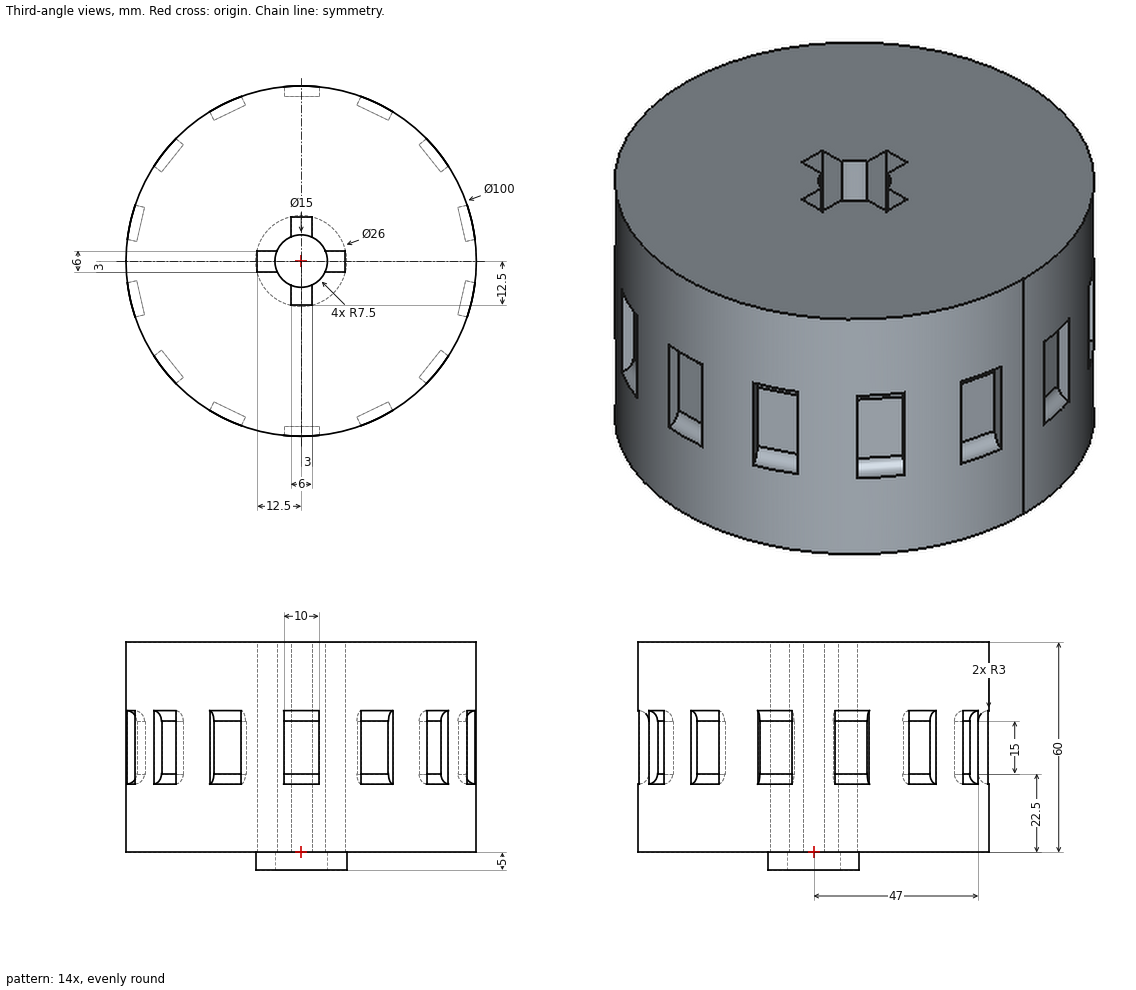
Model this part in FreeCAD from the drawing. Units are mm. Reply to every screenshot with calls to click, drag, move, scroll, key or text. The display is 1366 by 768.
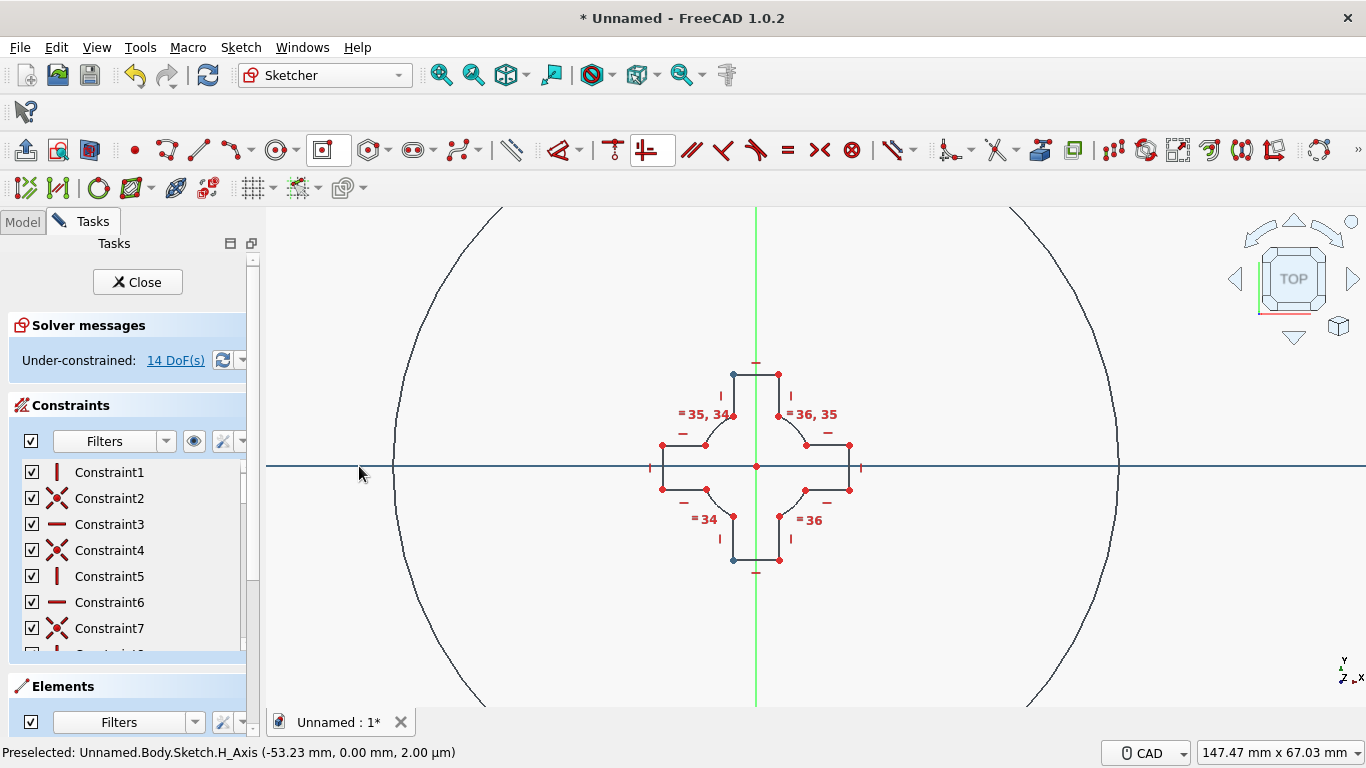
click(820, 150)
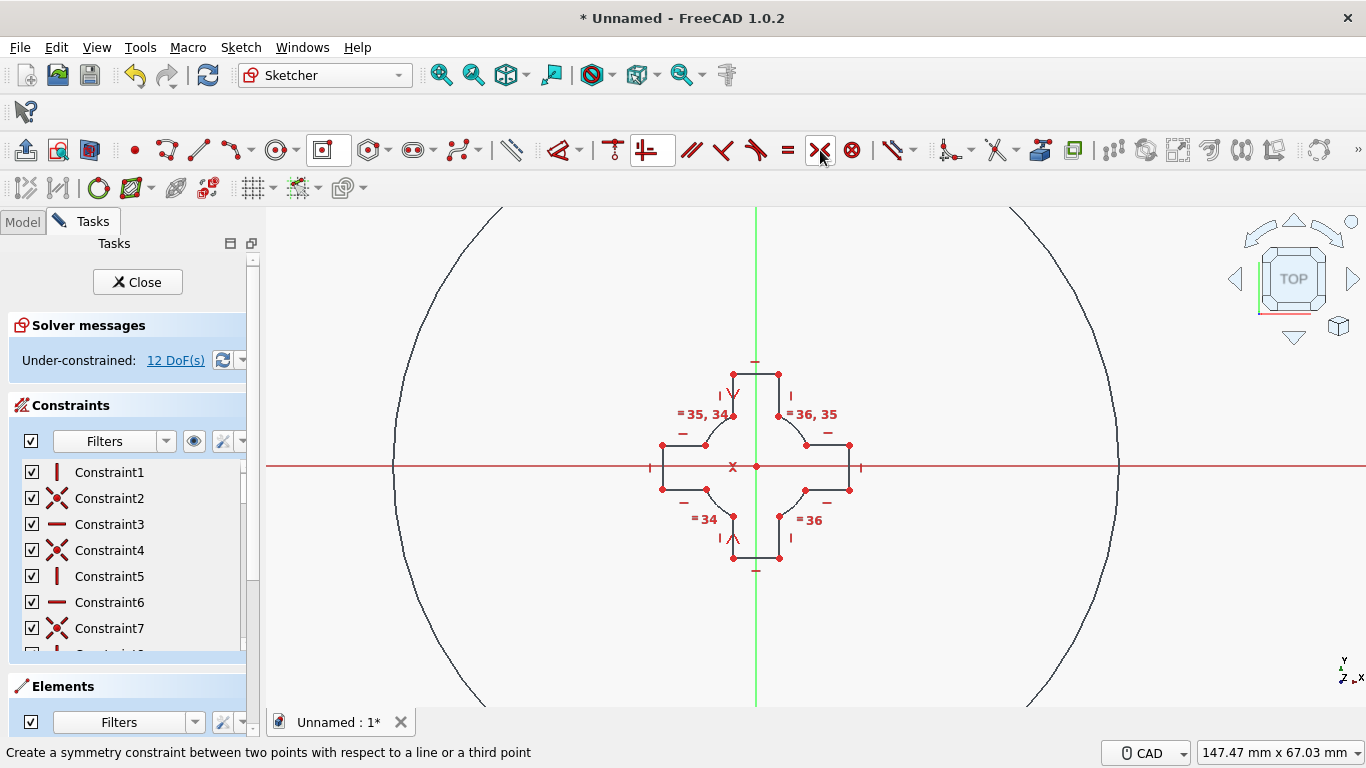
click(663, 446)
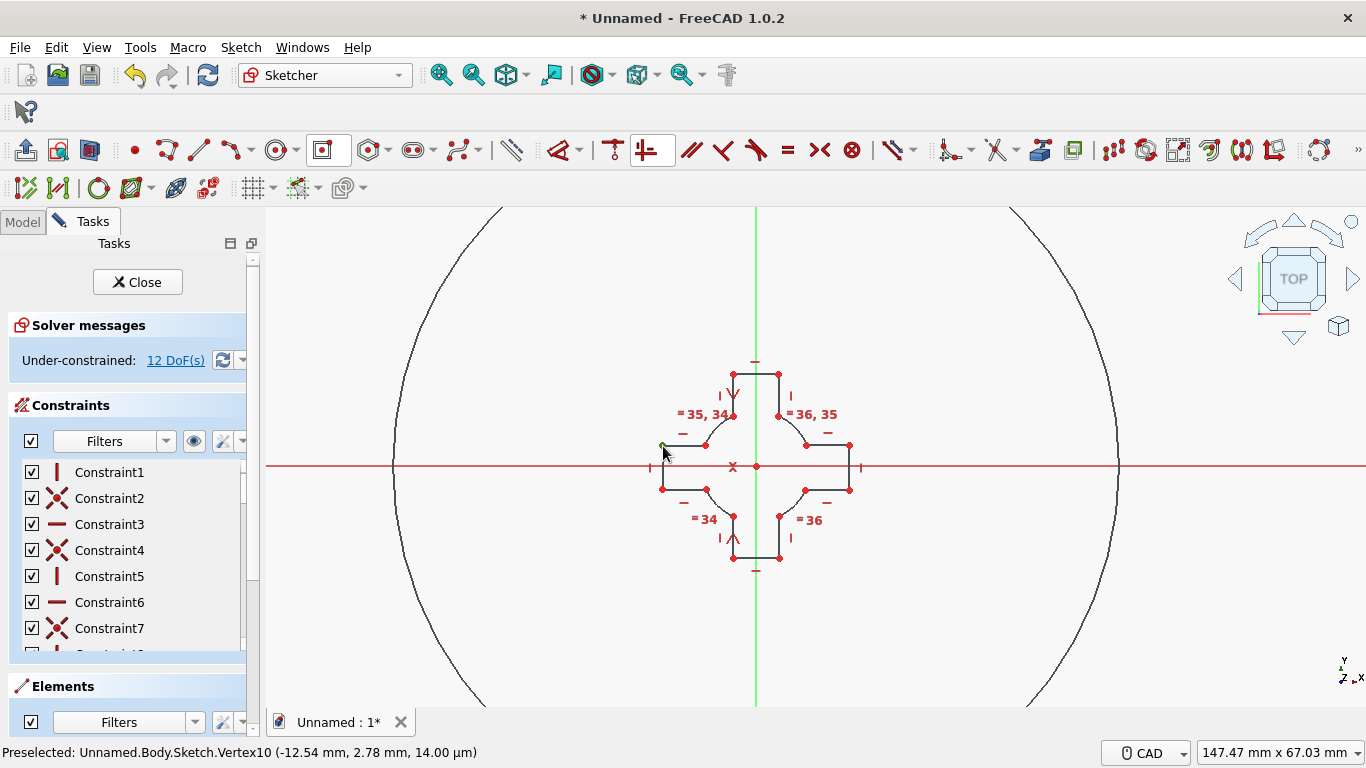
click(849, 445)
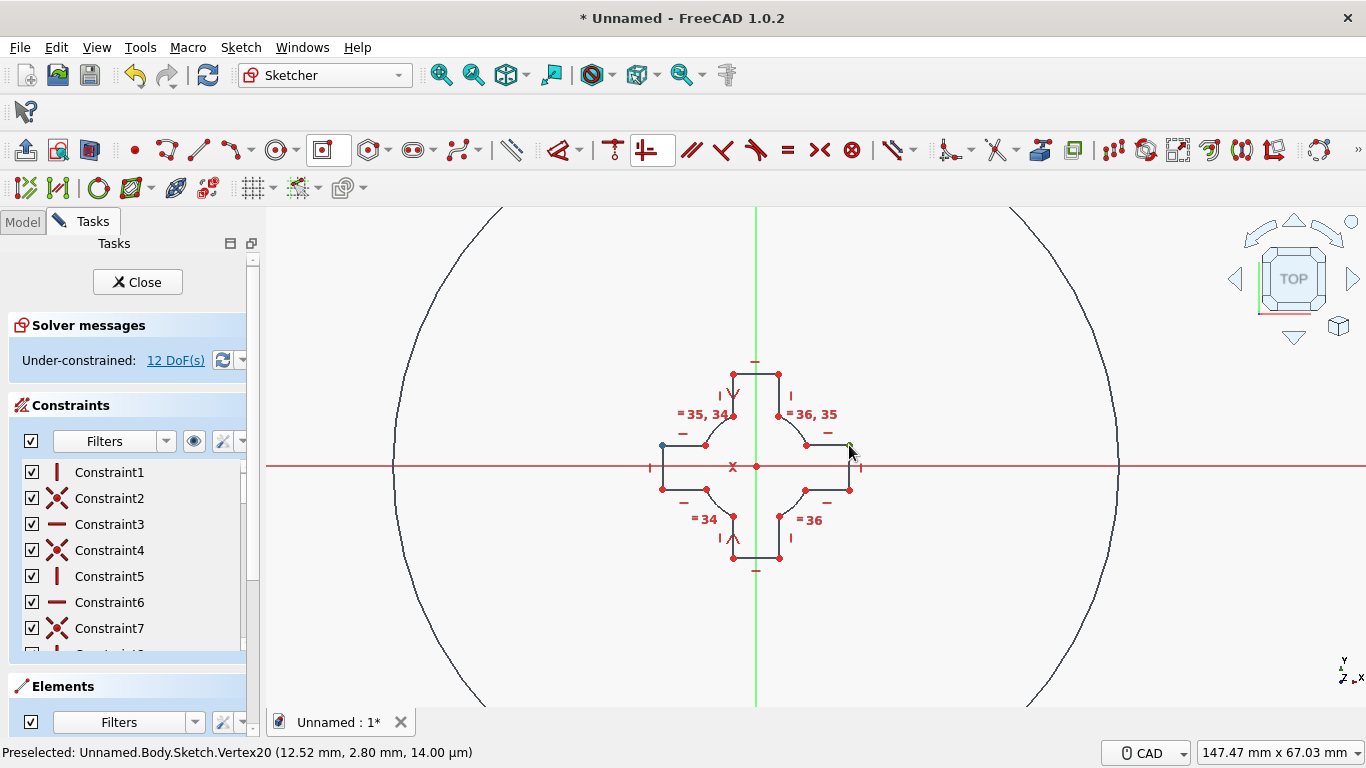
click(756, 647)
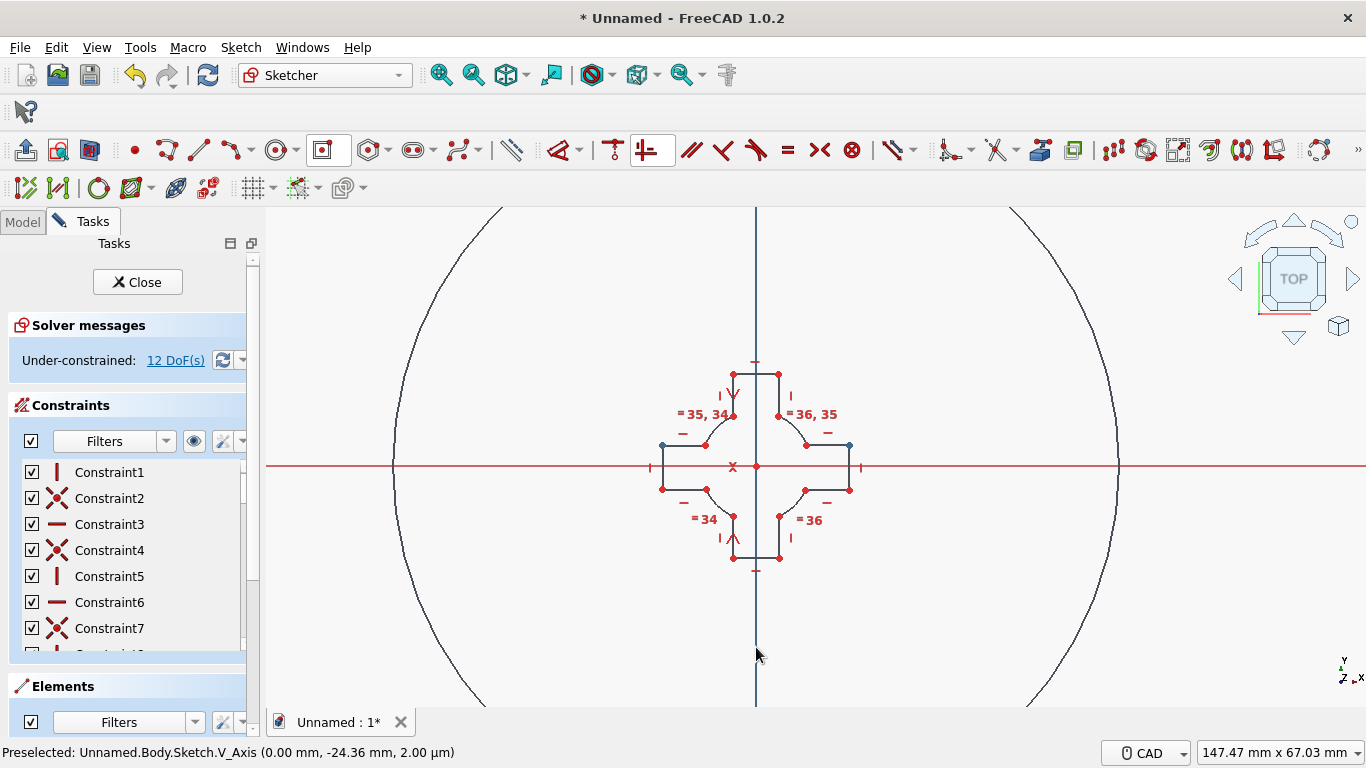
key(s)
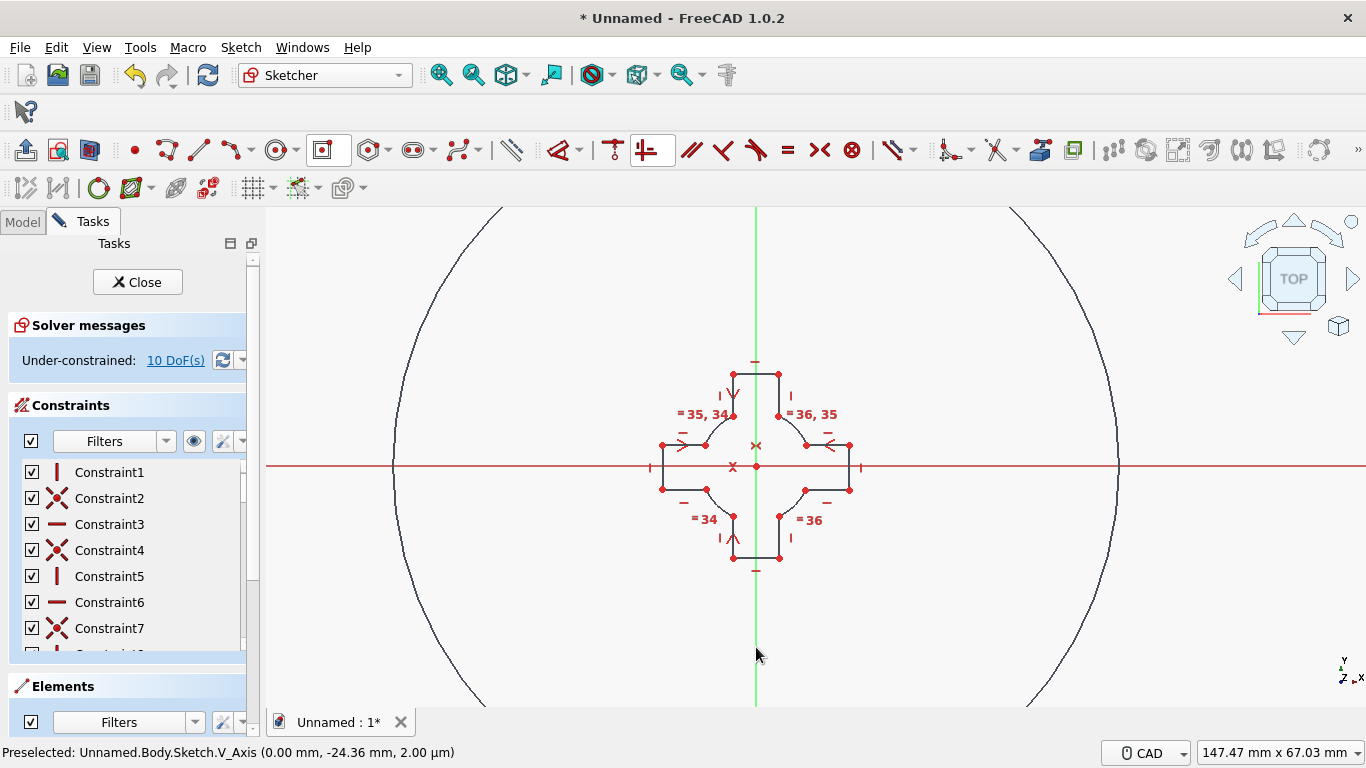
key(d)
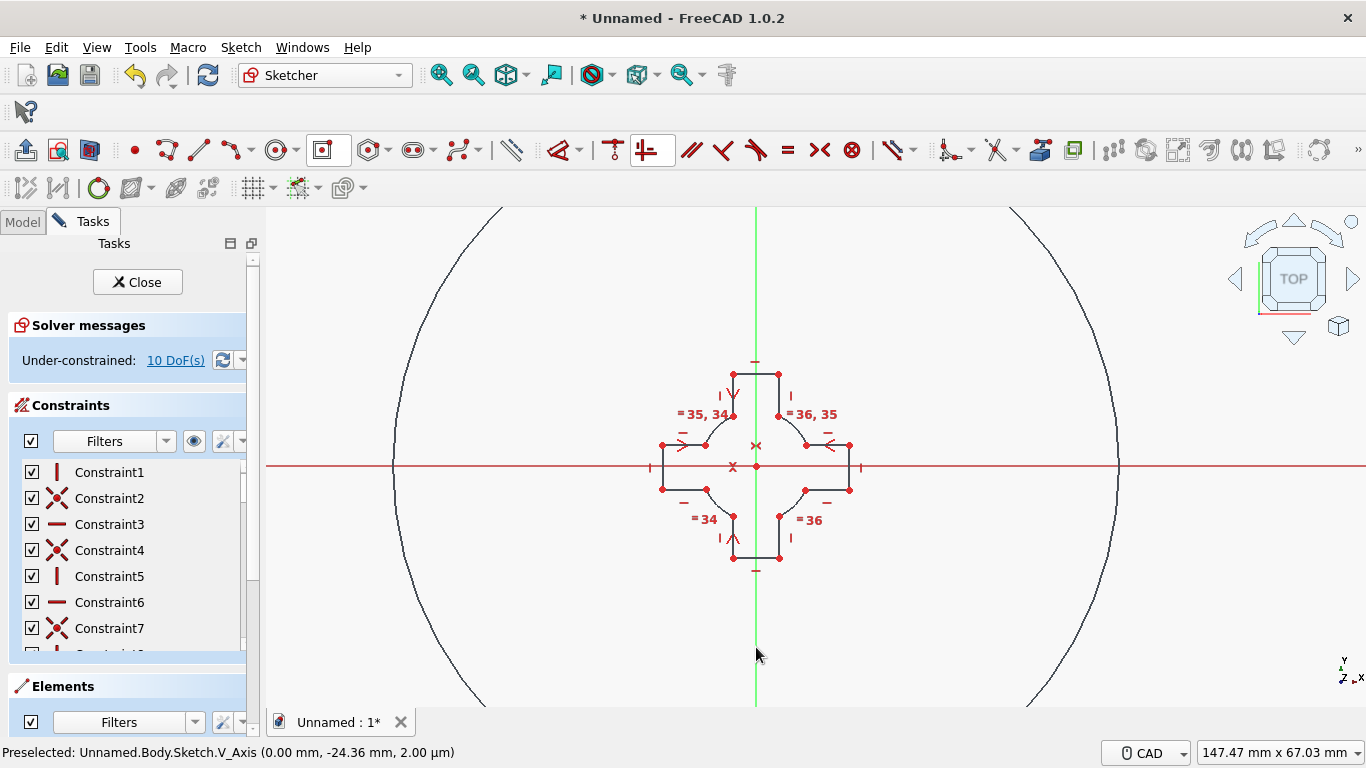
click(712, 500)
click(687, 519)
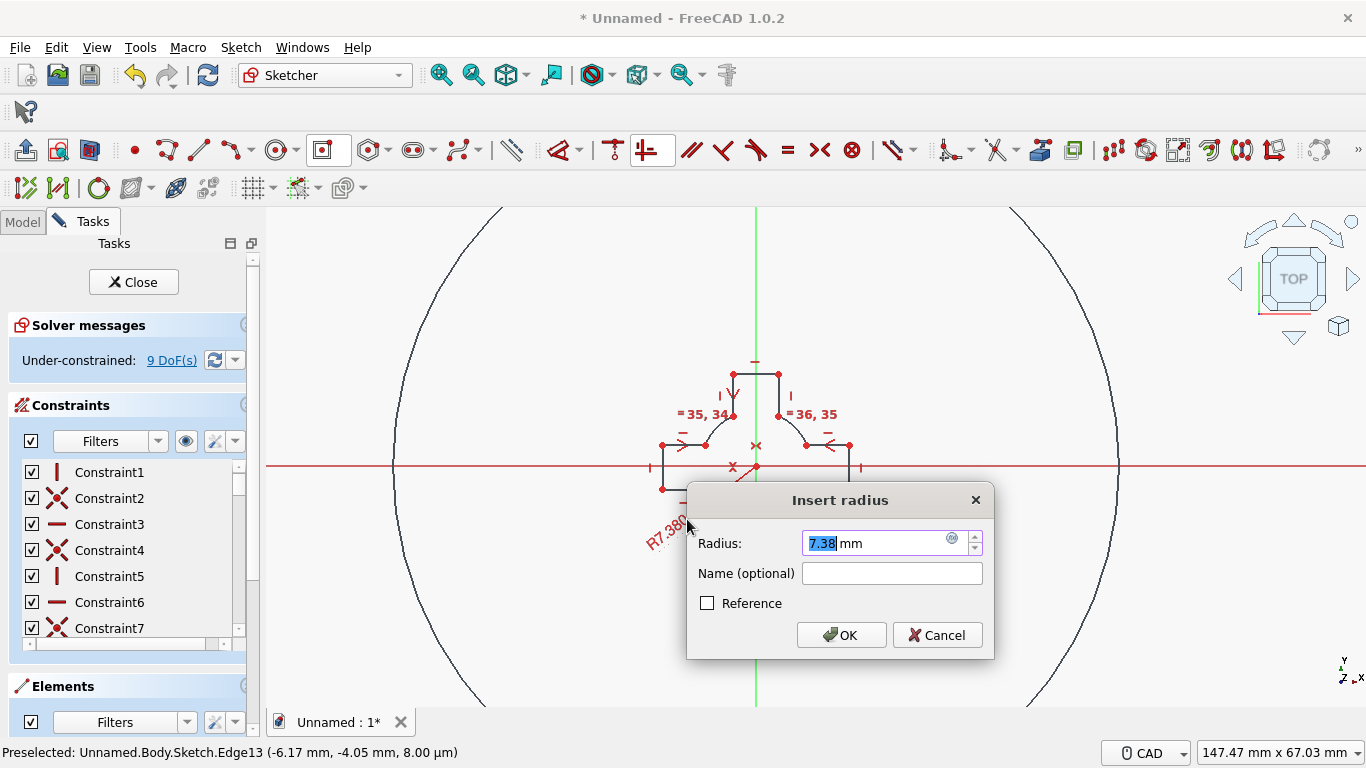
text(7.5)
key(Return)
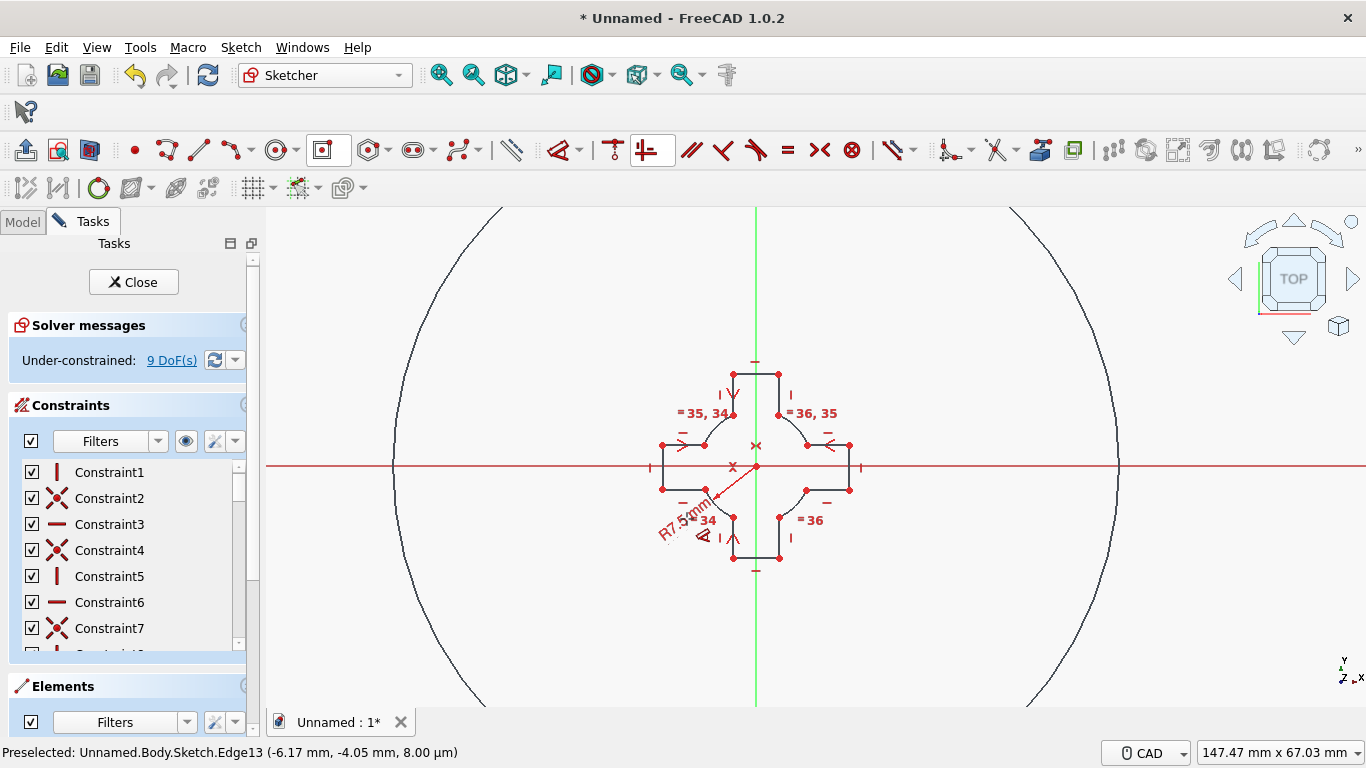
scroll(393, 456, up, 2)